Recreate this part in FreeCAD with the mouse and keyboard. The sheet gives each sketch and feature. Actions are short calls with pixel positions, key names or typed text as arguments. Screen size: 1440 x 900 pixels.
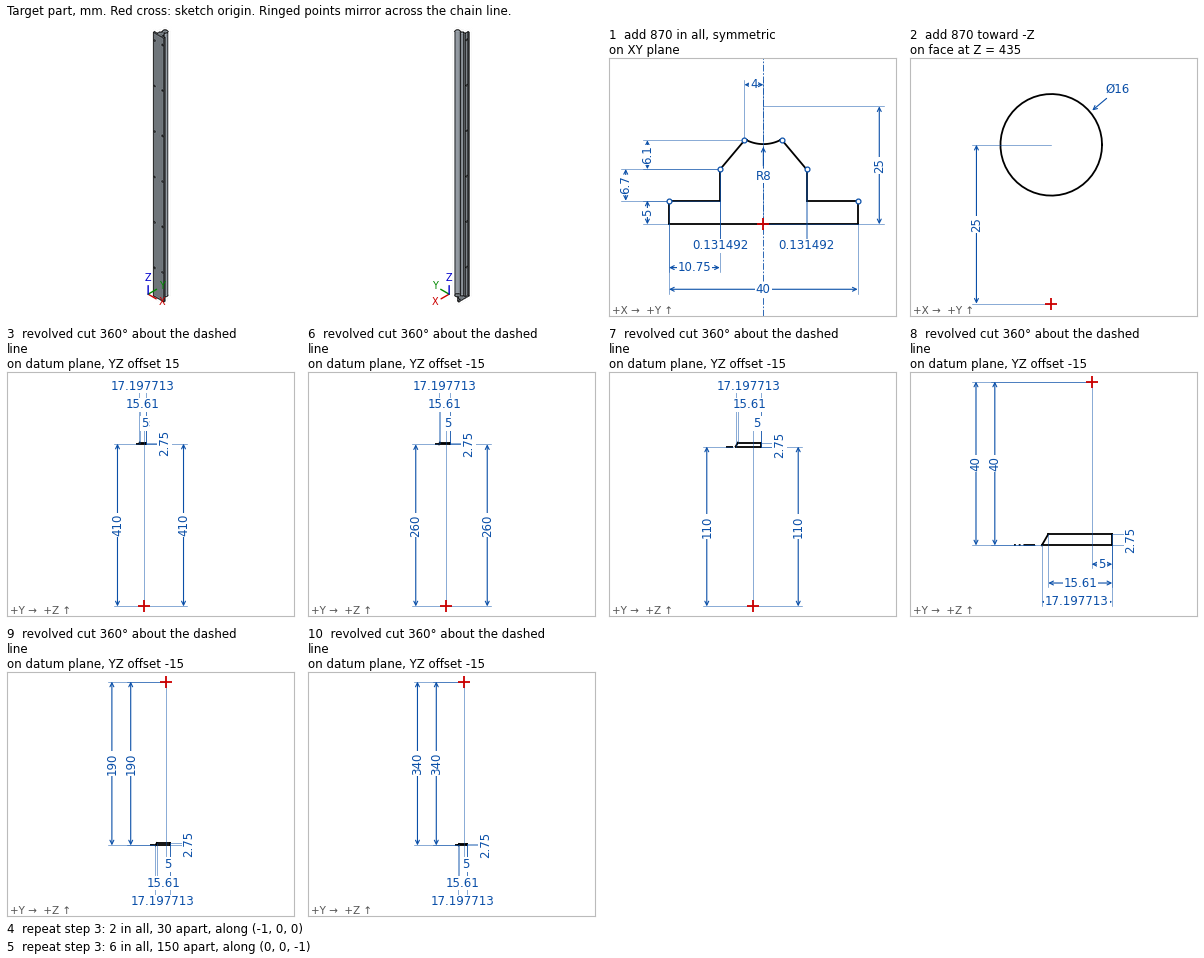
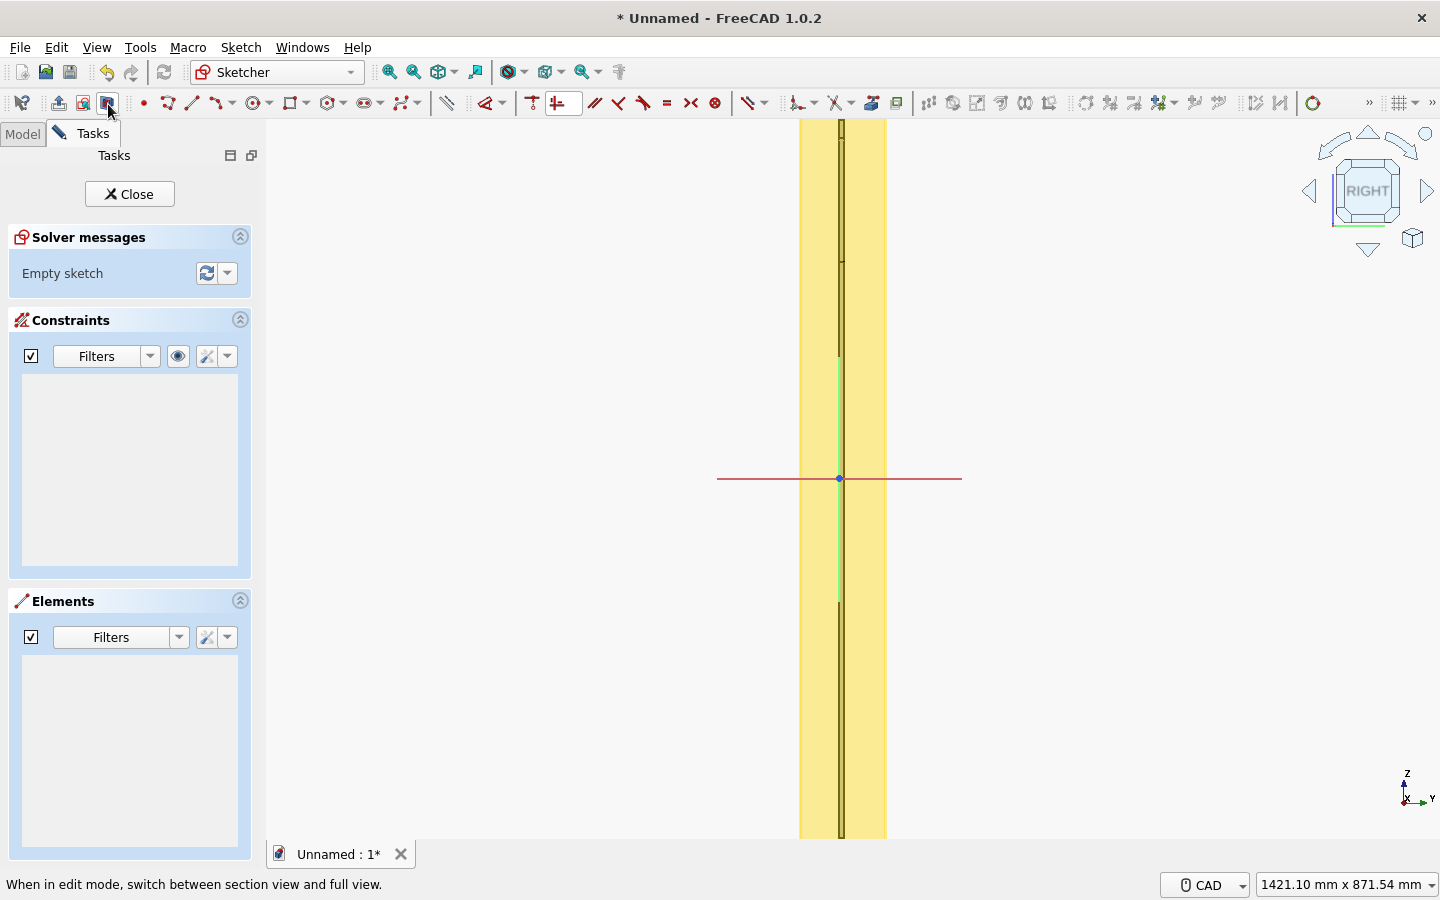
scroll(836, 382, up, 15)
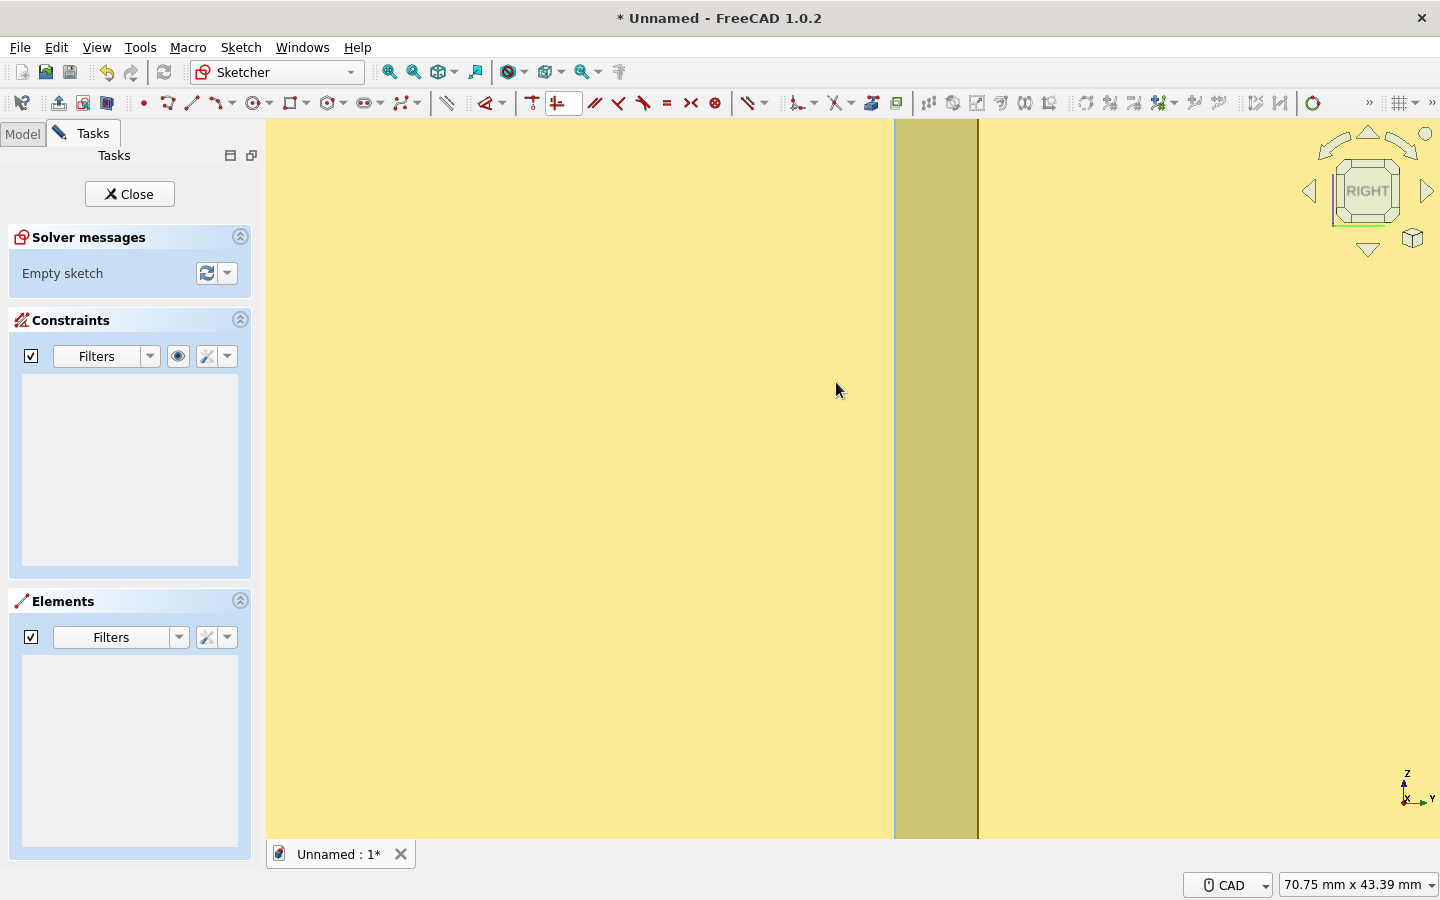
scroll(770, 471, up, 3)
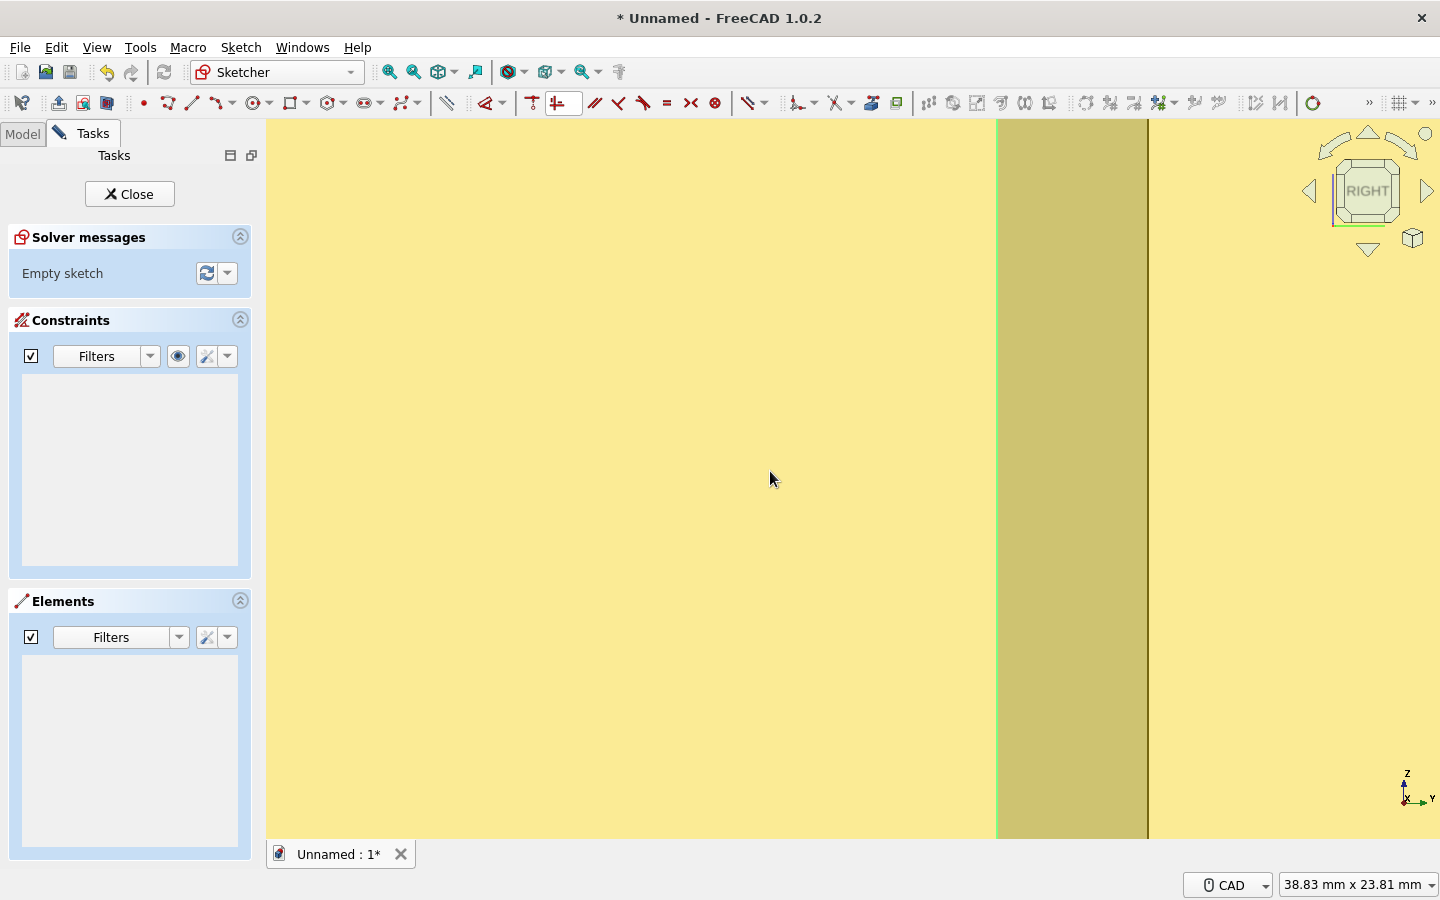
click(168, 104)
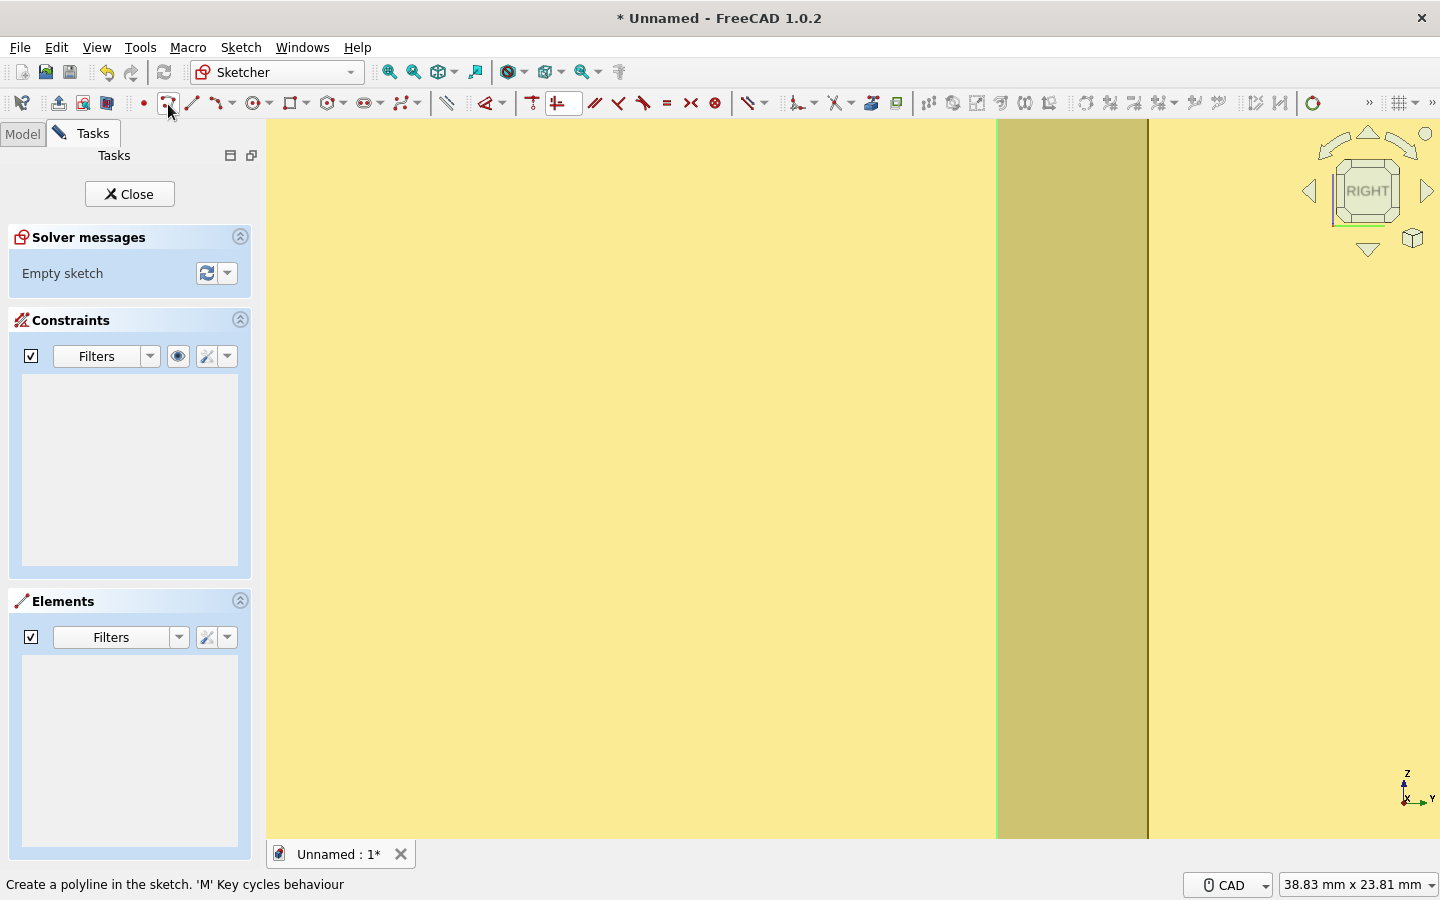
click(1148, 520)
click(1148, 437)
click(676, 437)
click(628, 520)
click(1148, 521)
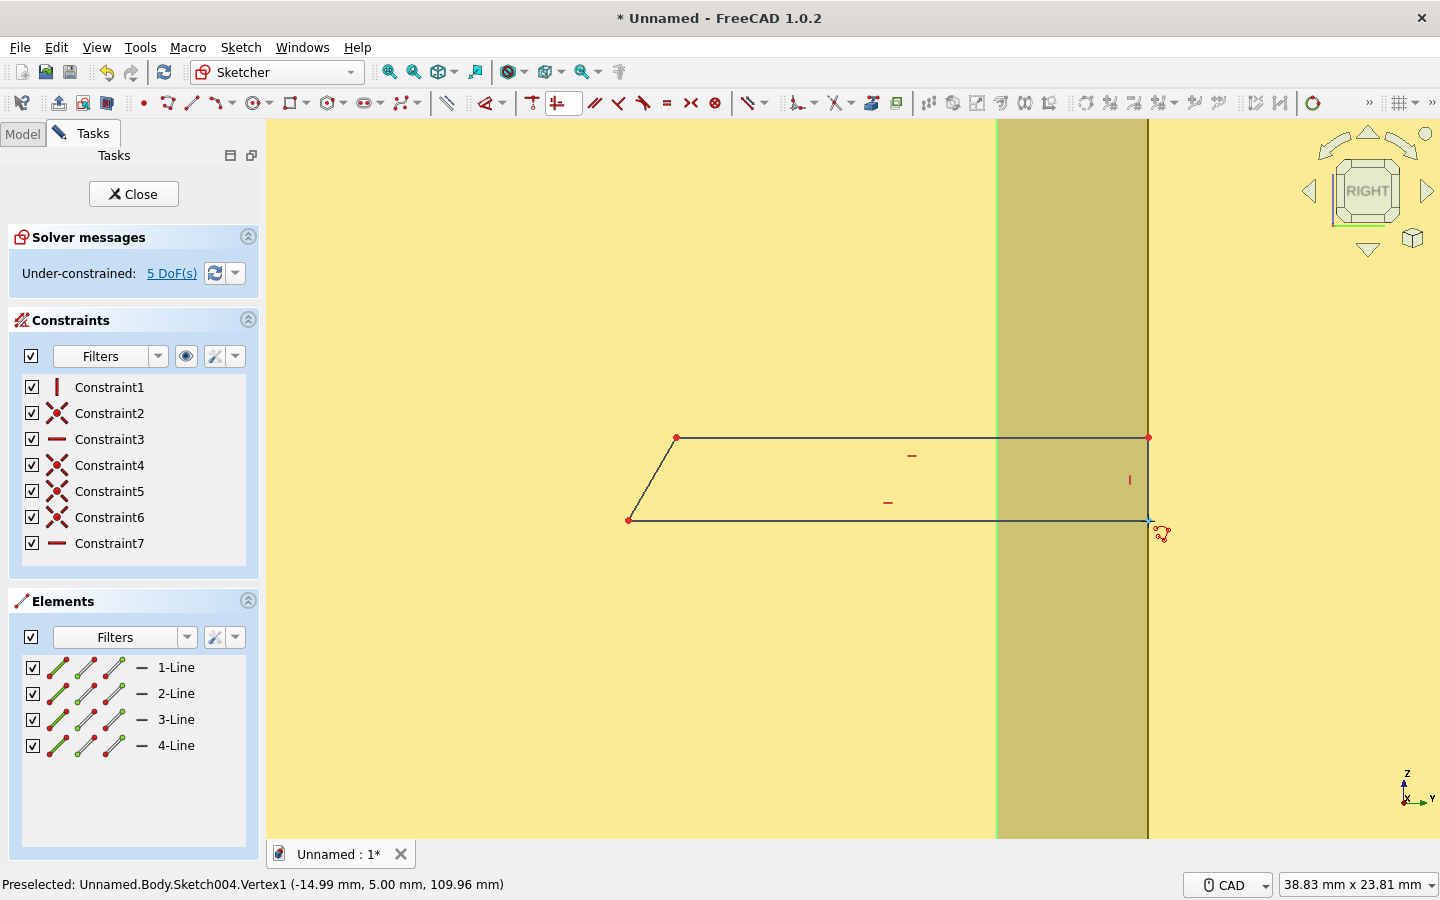
click(192, 104)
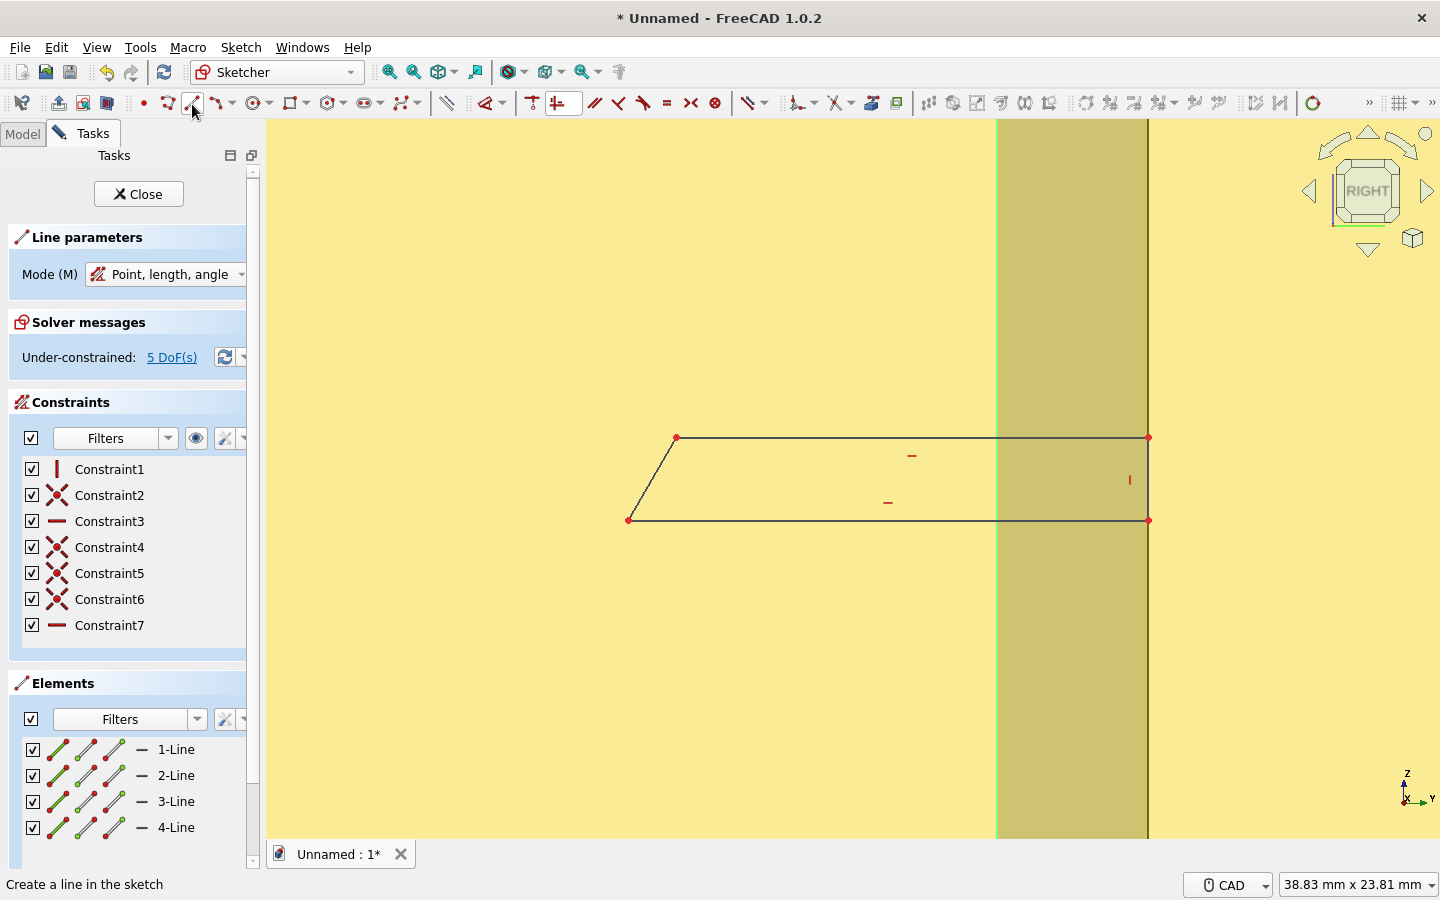
click(576, 520)
click(420, 520)
key(Escape)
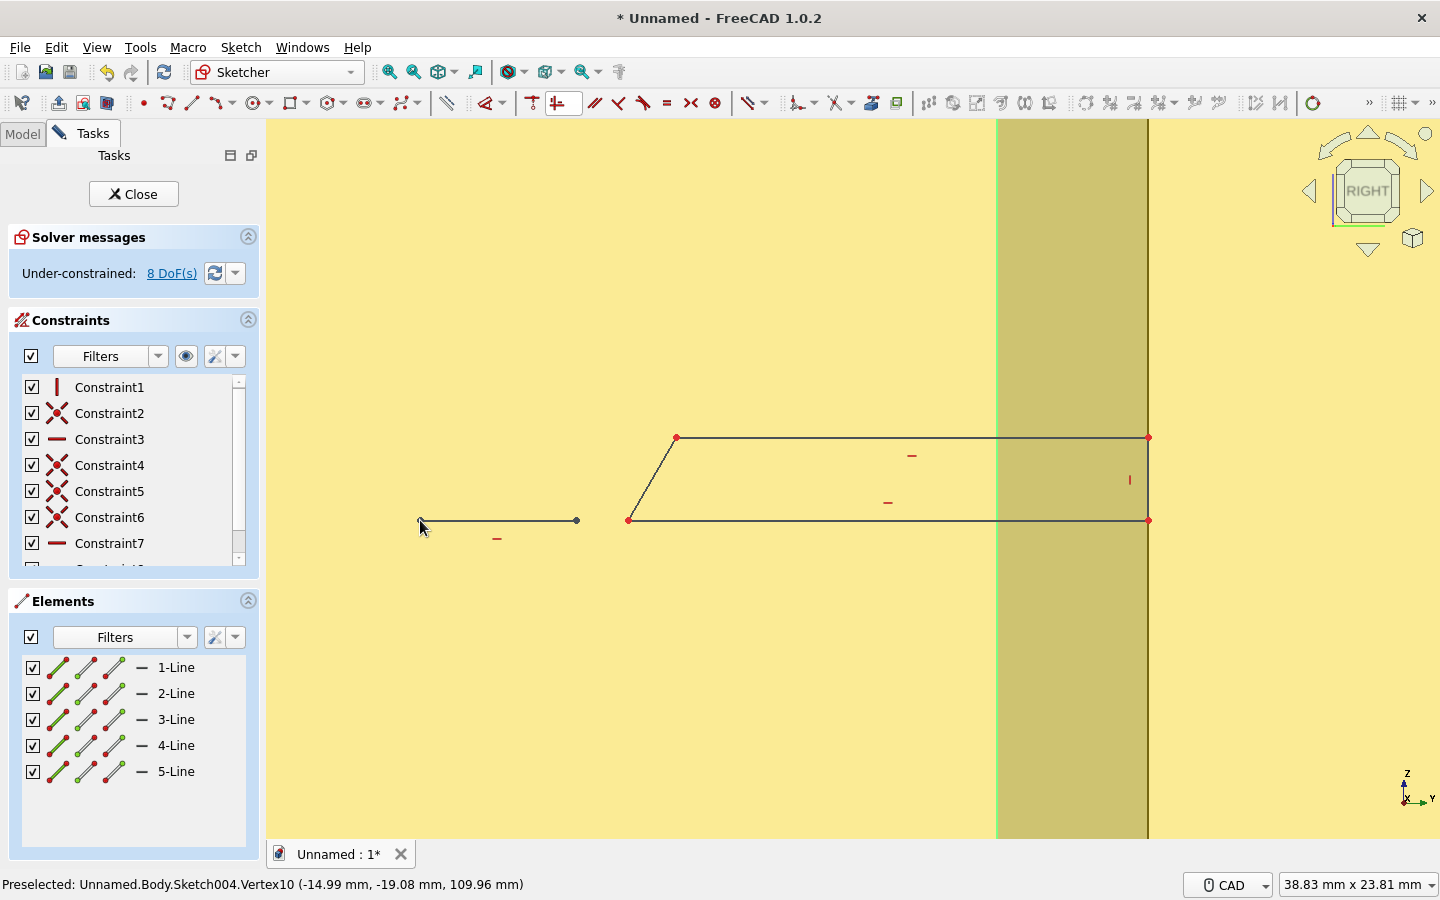
click(529, 521)